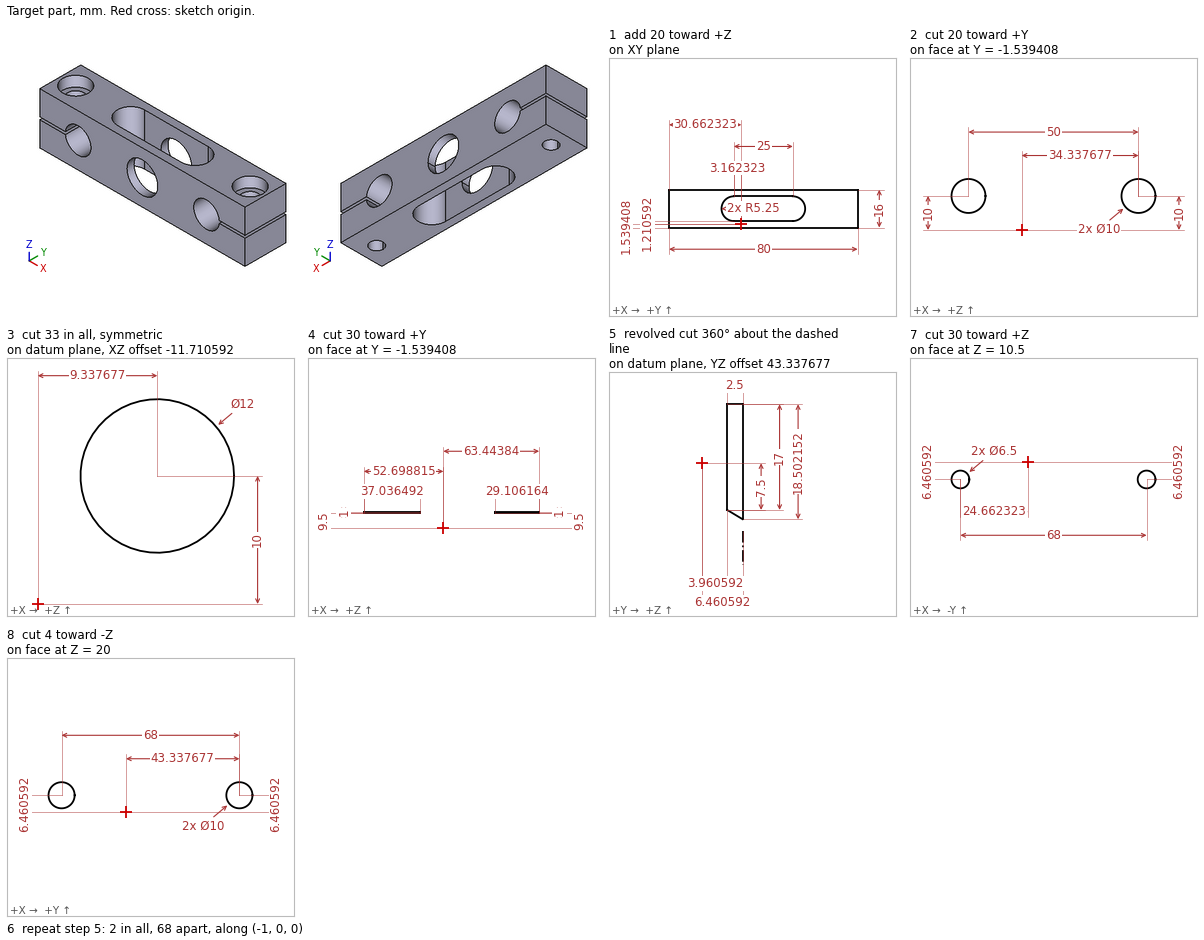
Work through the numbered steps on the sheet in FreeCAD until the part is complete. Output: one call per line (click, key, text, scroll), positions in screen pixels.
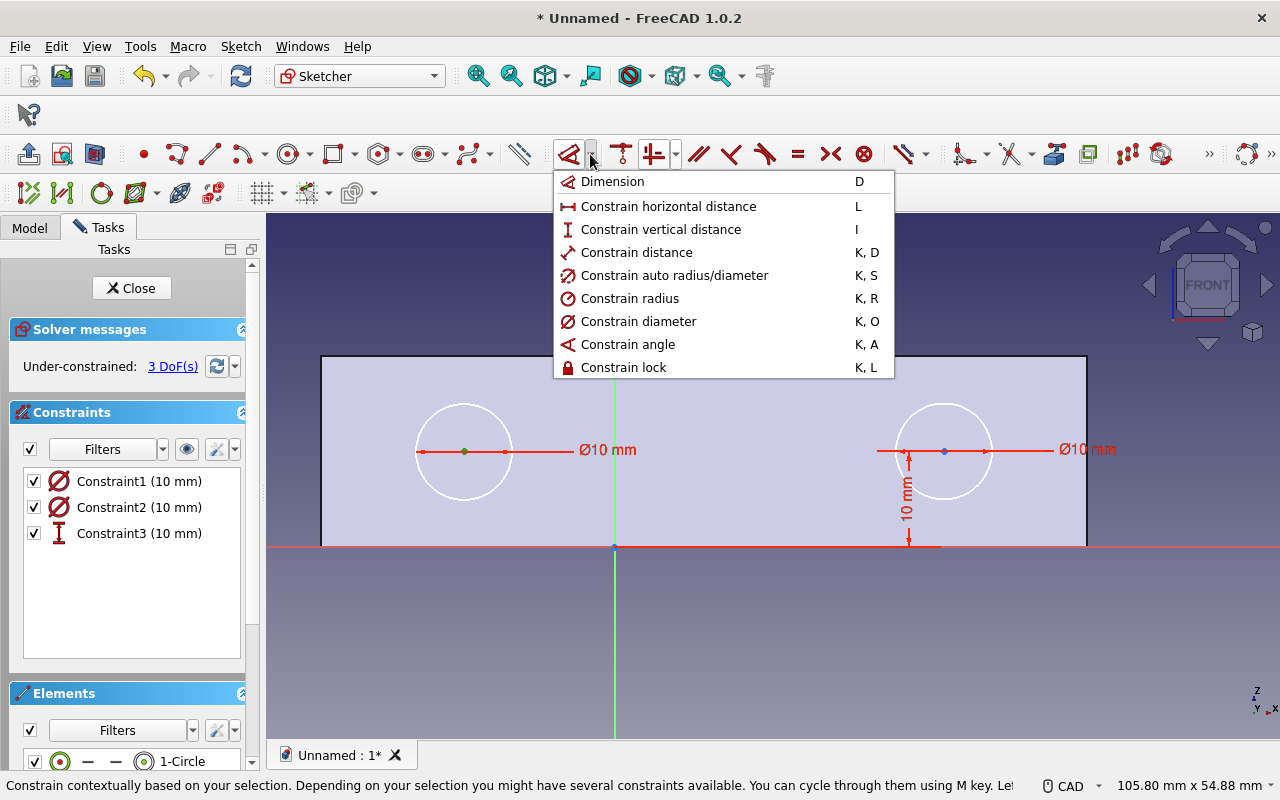
click(724, 230)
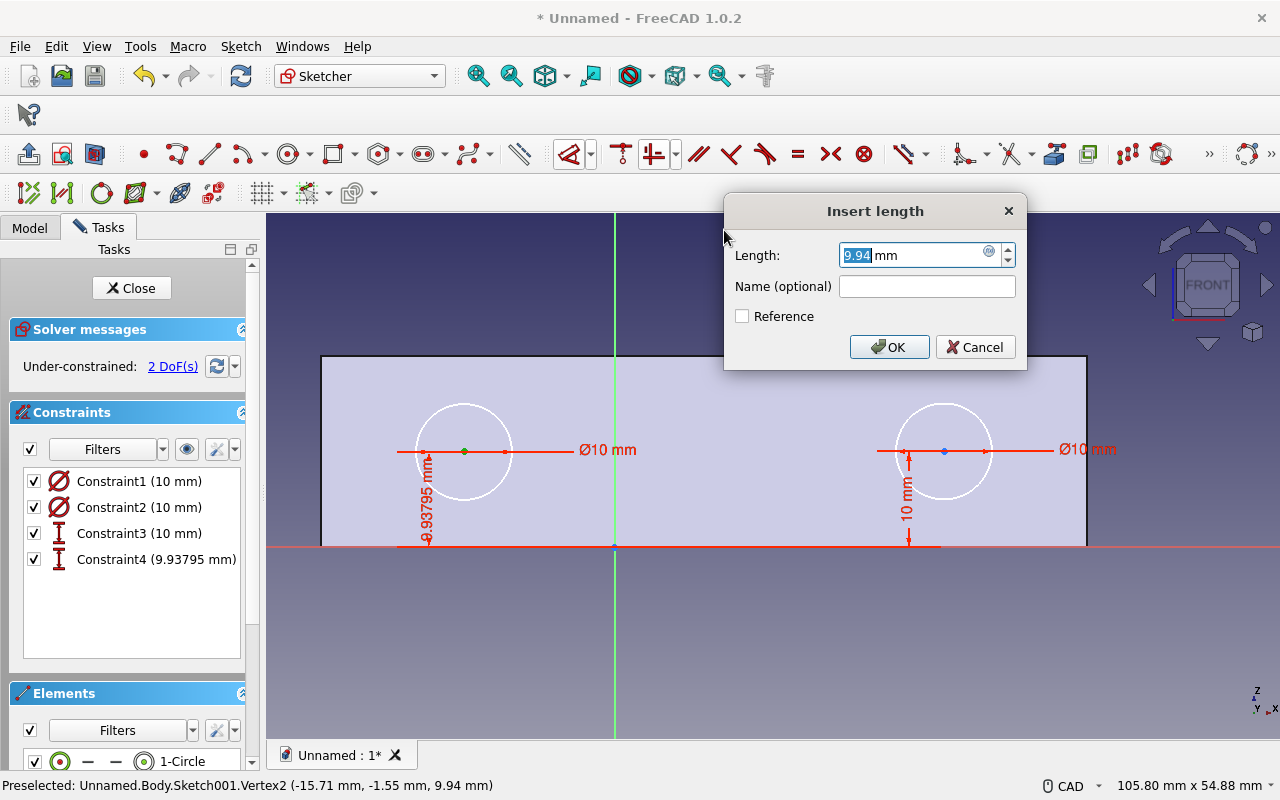
text(10)
key(Return)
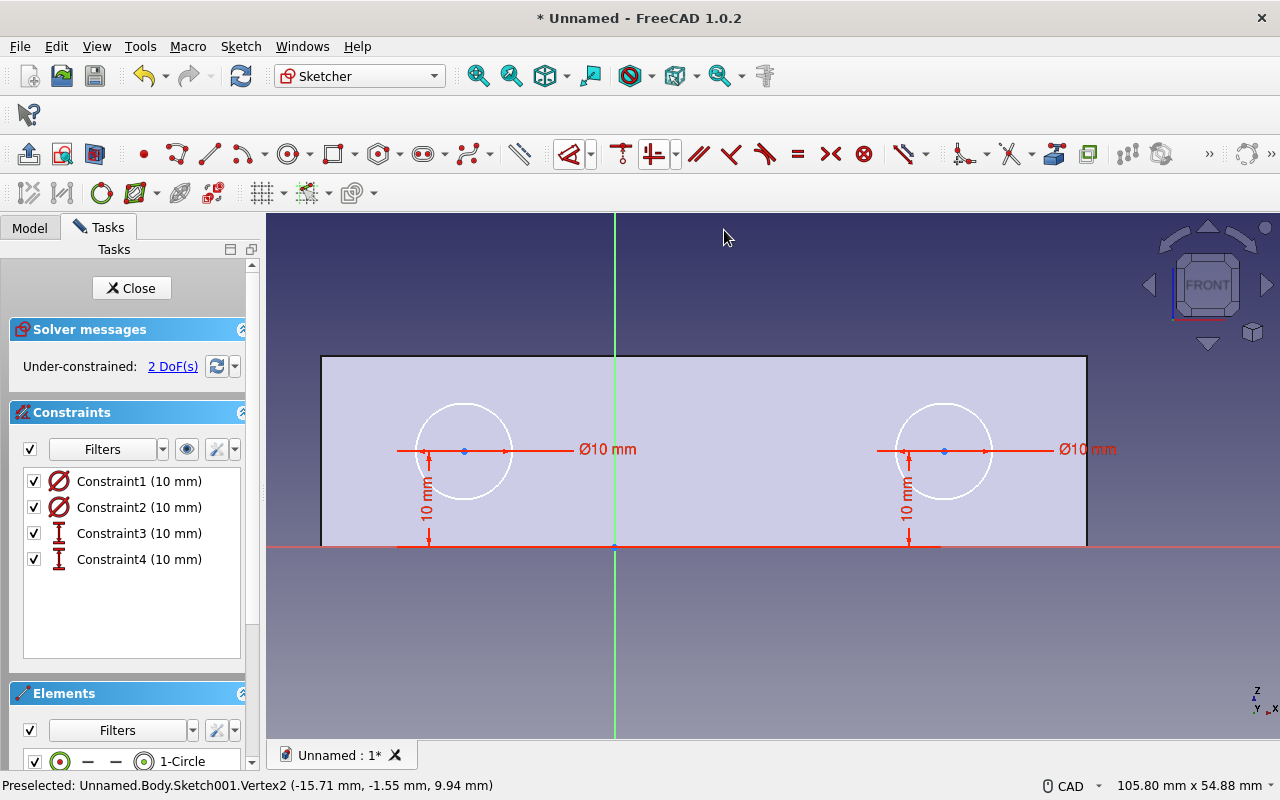
click(944, 451)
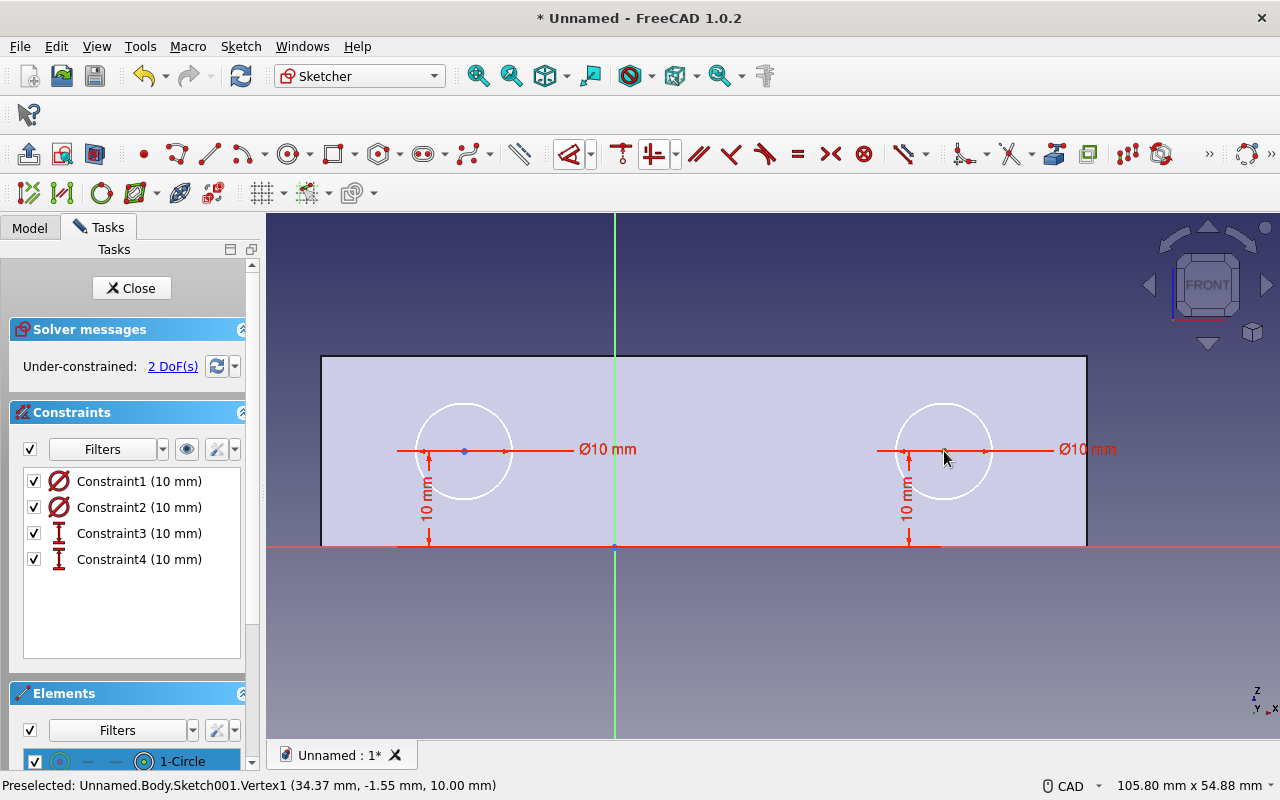
click(464, 451)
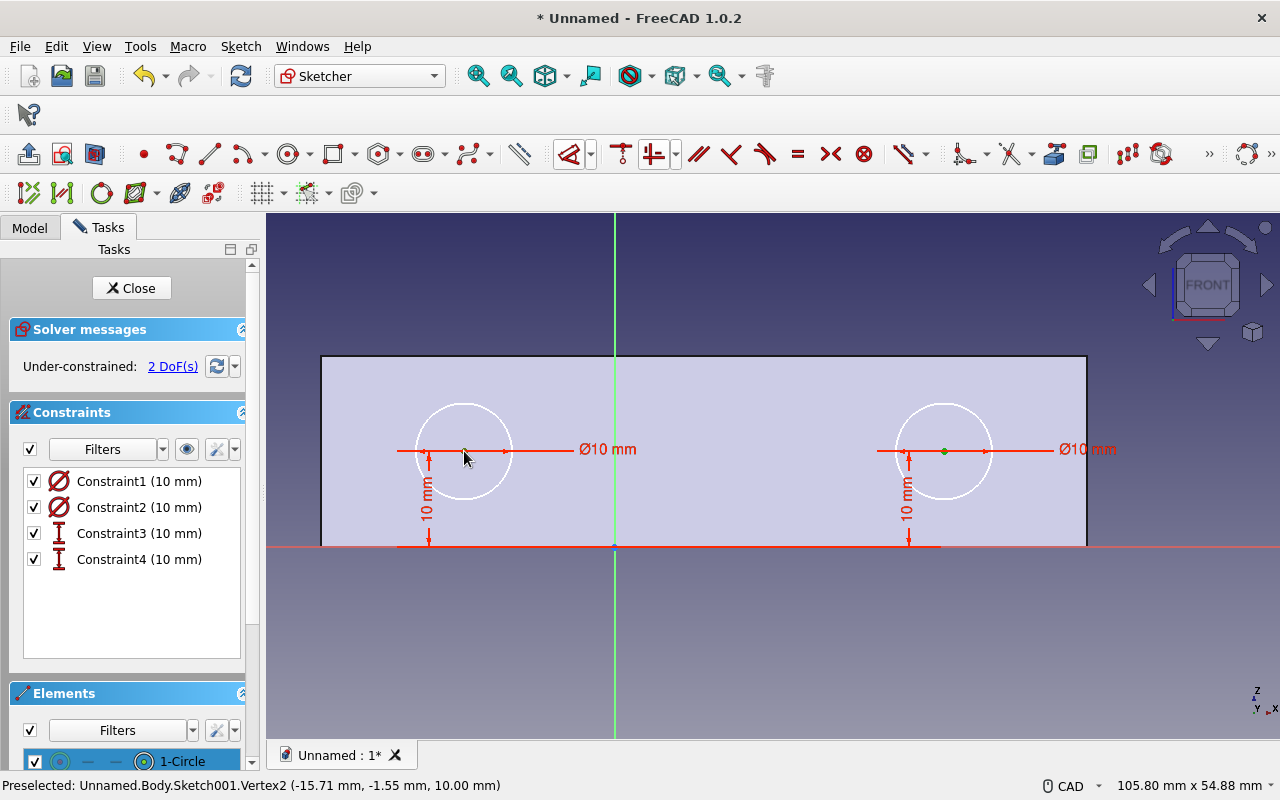
key(l)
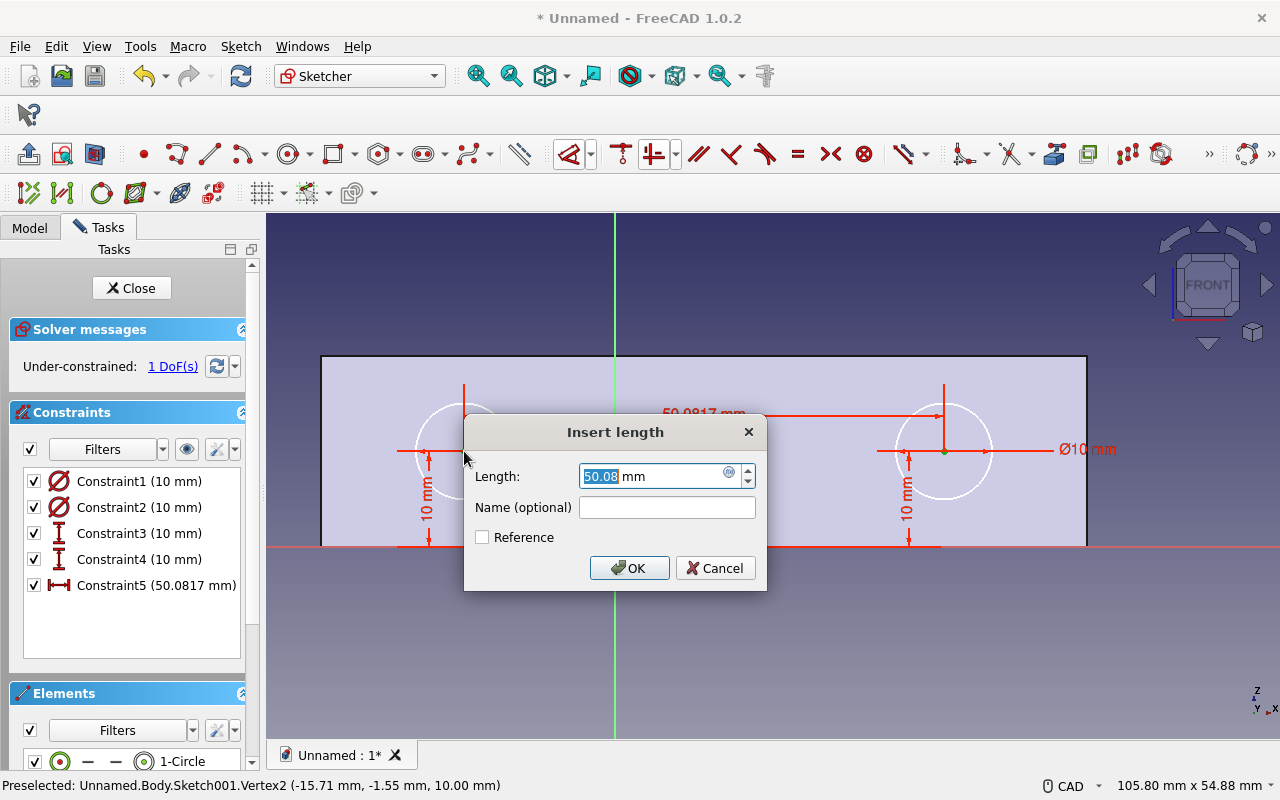
text(50)
key(Return)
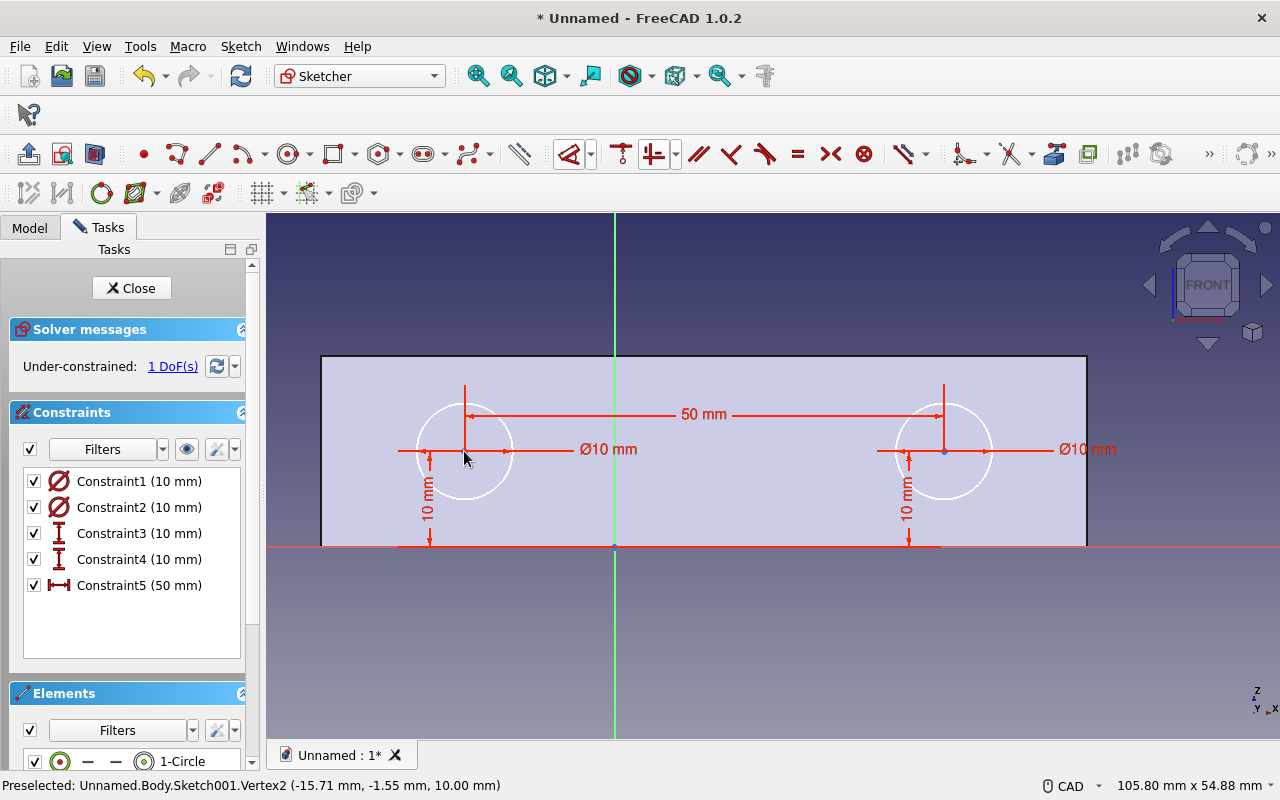
click(944, 451)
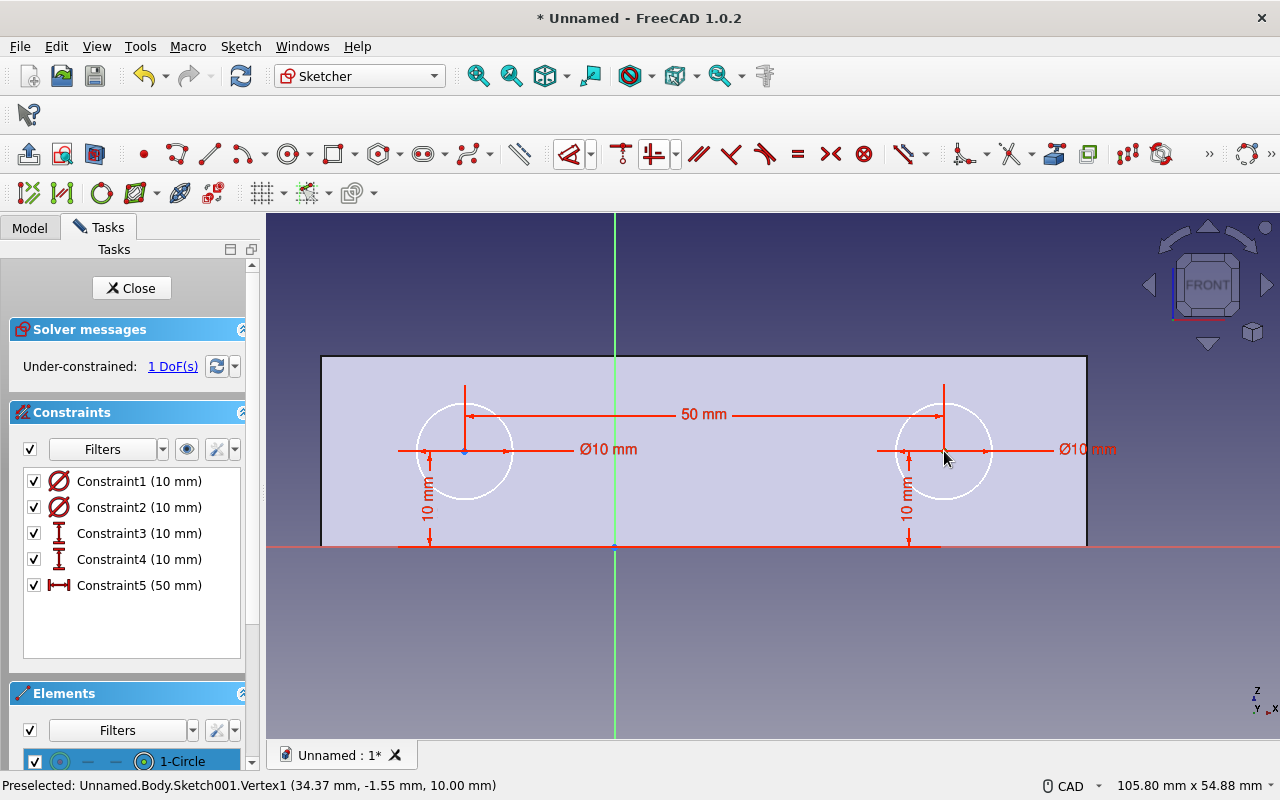
key(l)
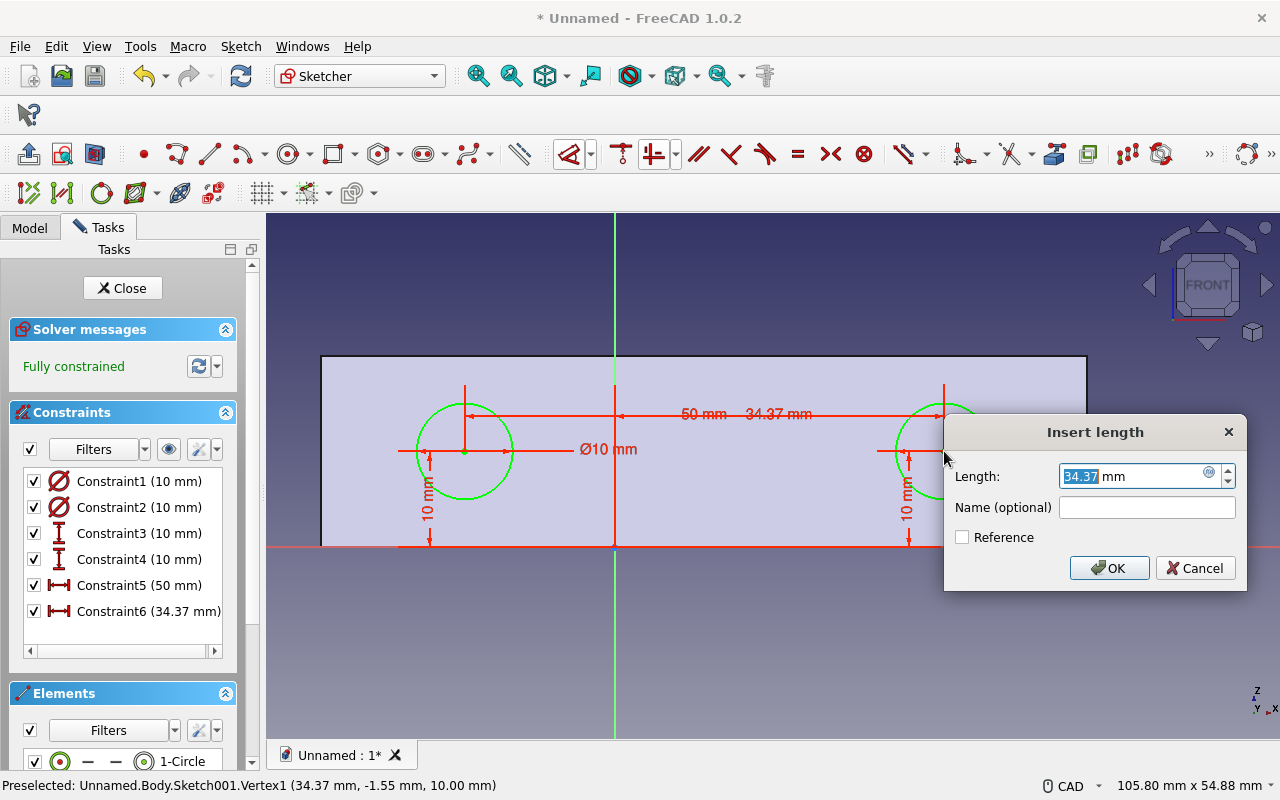
text(34.337677)
key(Return)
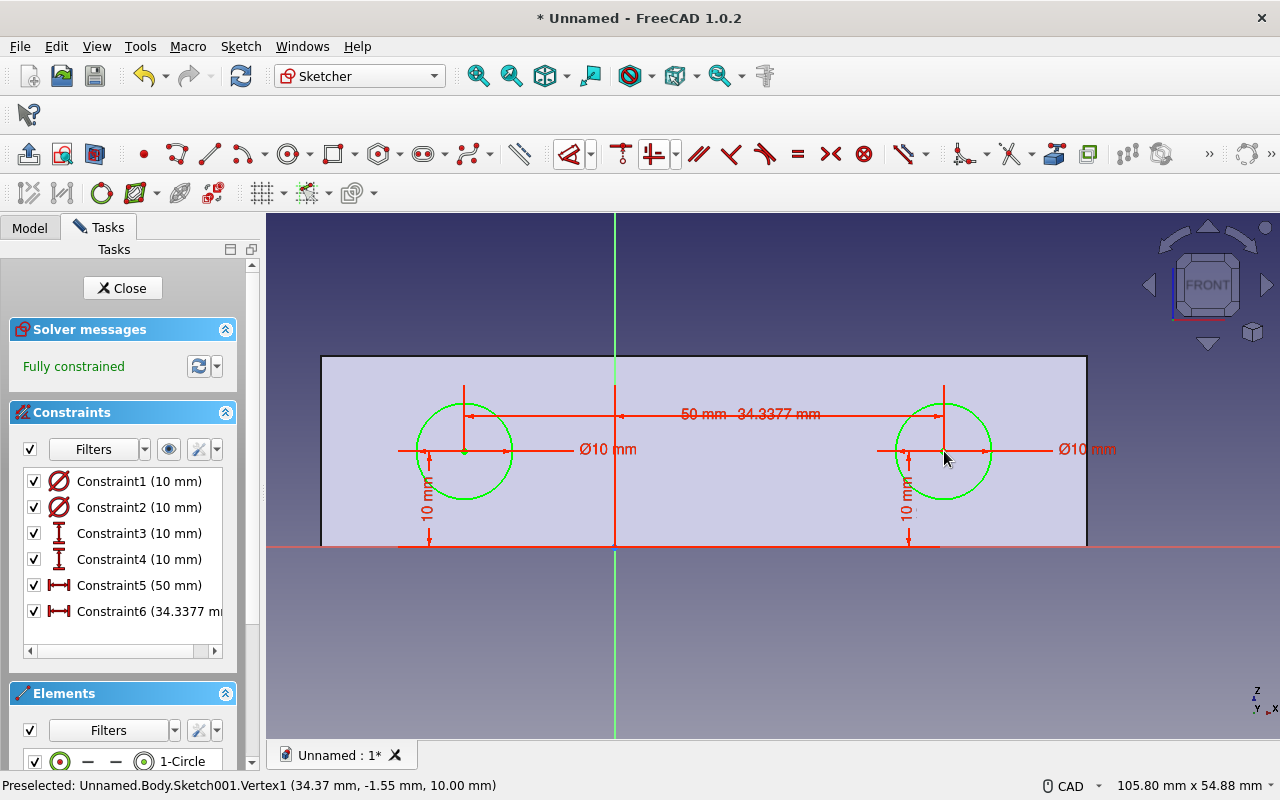
click(123, 288)